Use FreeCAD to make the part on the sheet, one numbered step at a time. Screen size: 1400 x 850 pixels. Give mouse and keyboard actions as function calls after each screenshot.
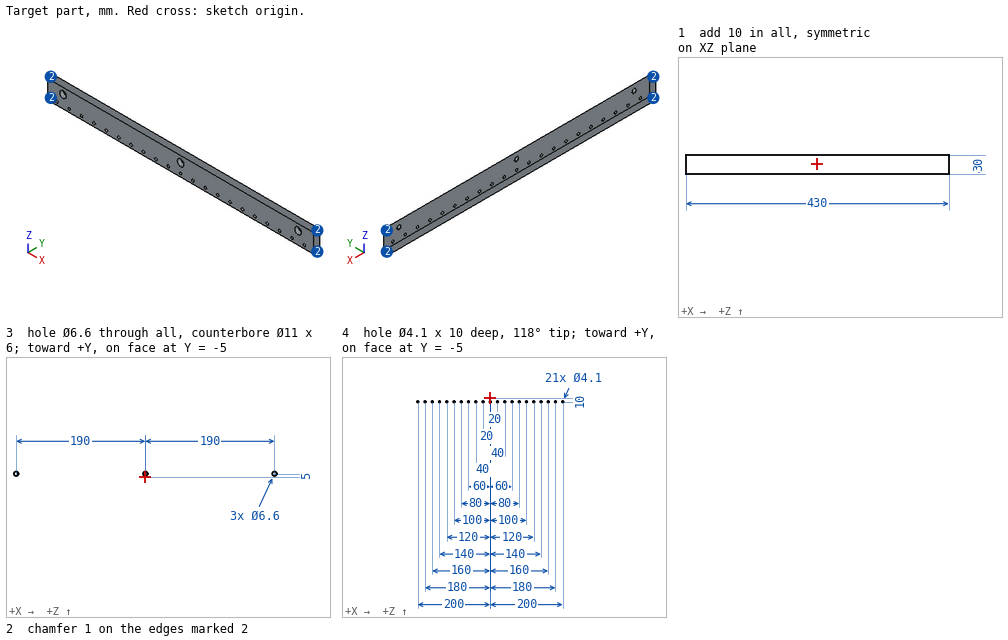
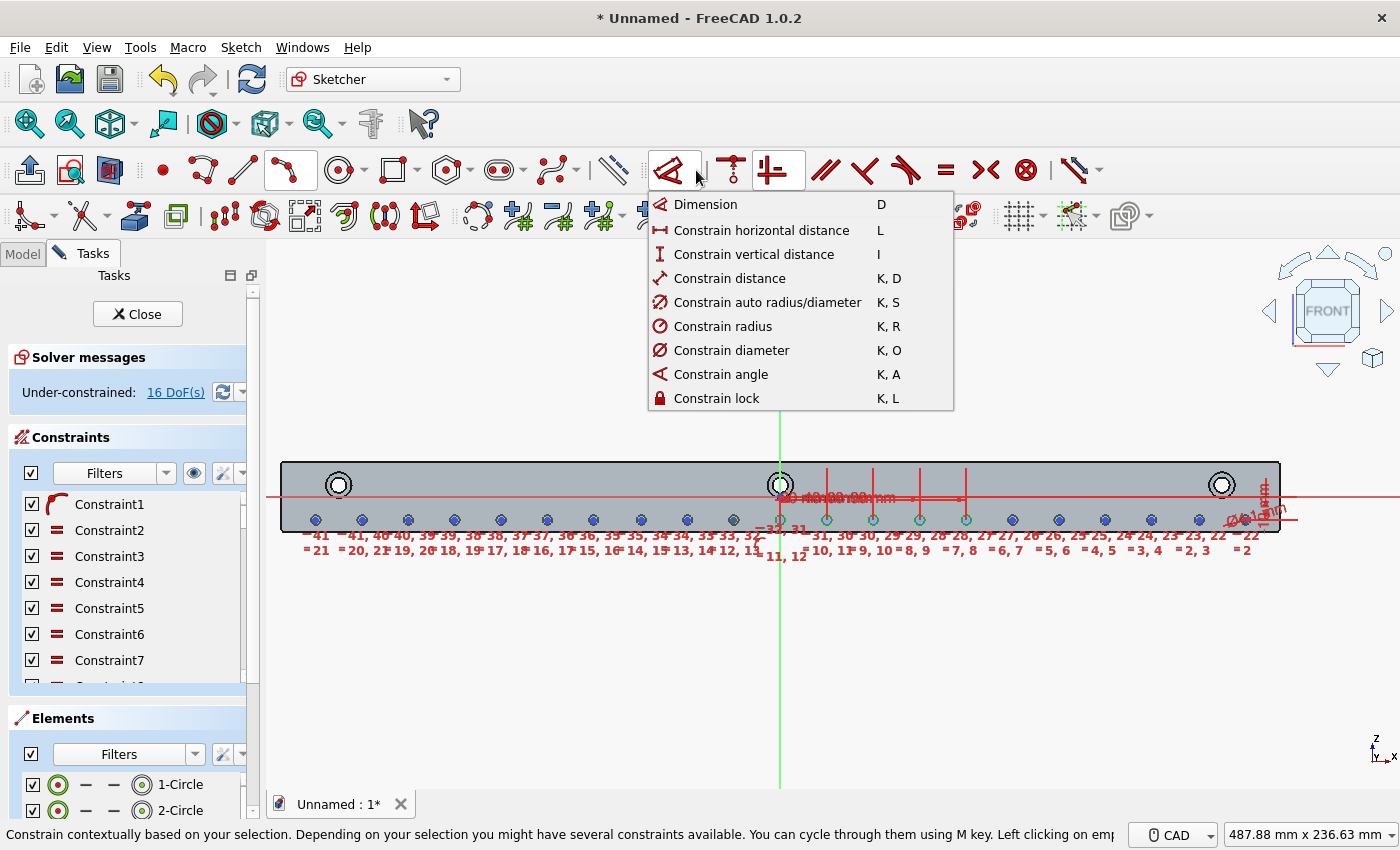
click(801, 230)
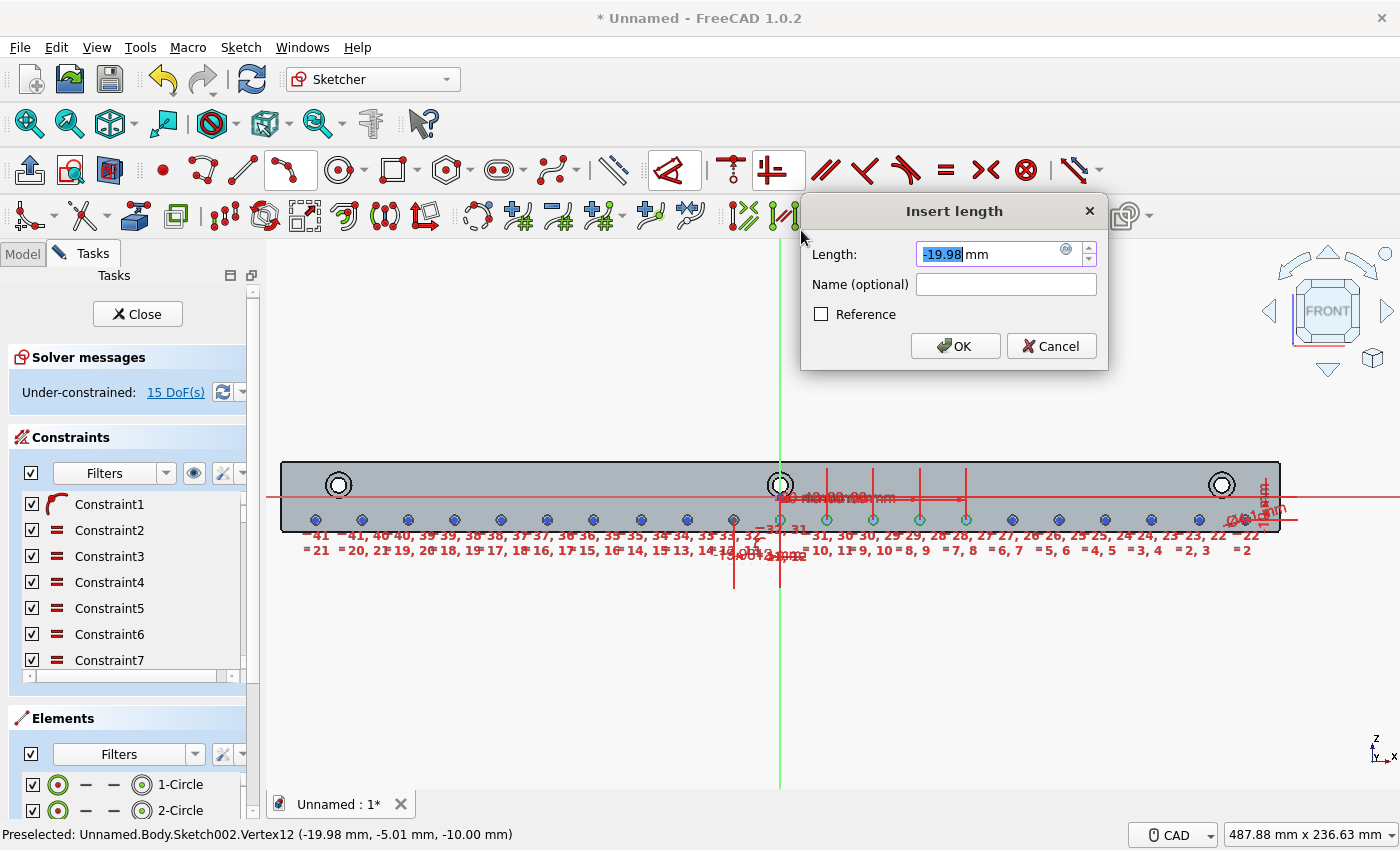
text(-20)
key(Return)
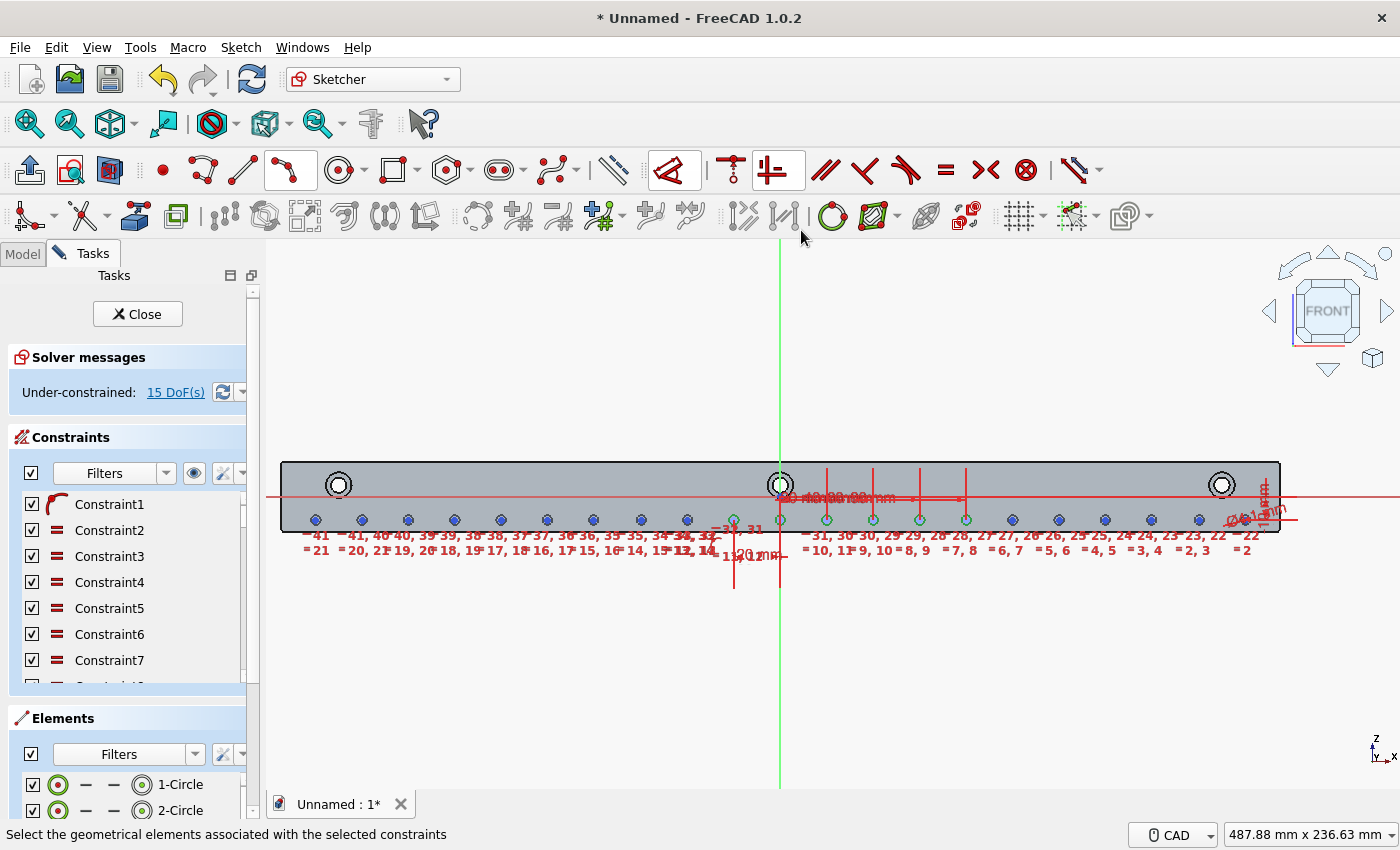
click(688, 520)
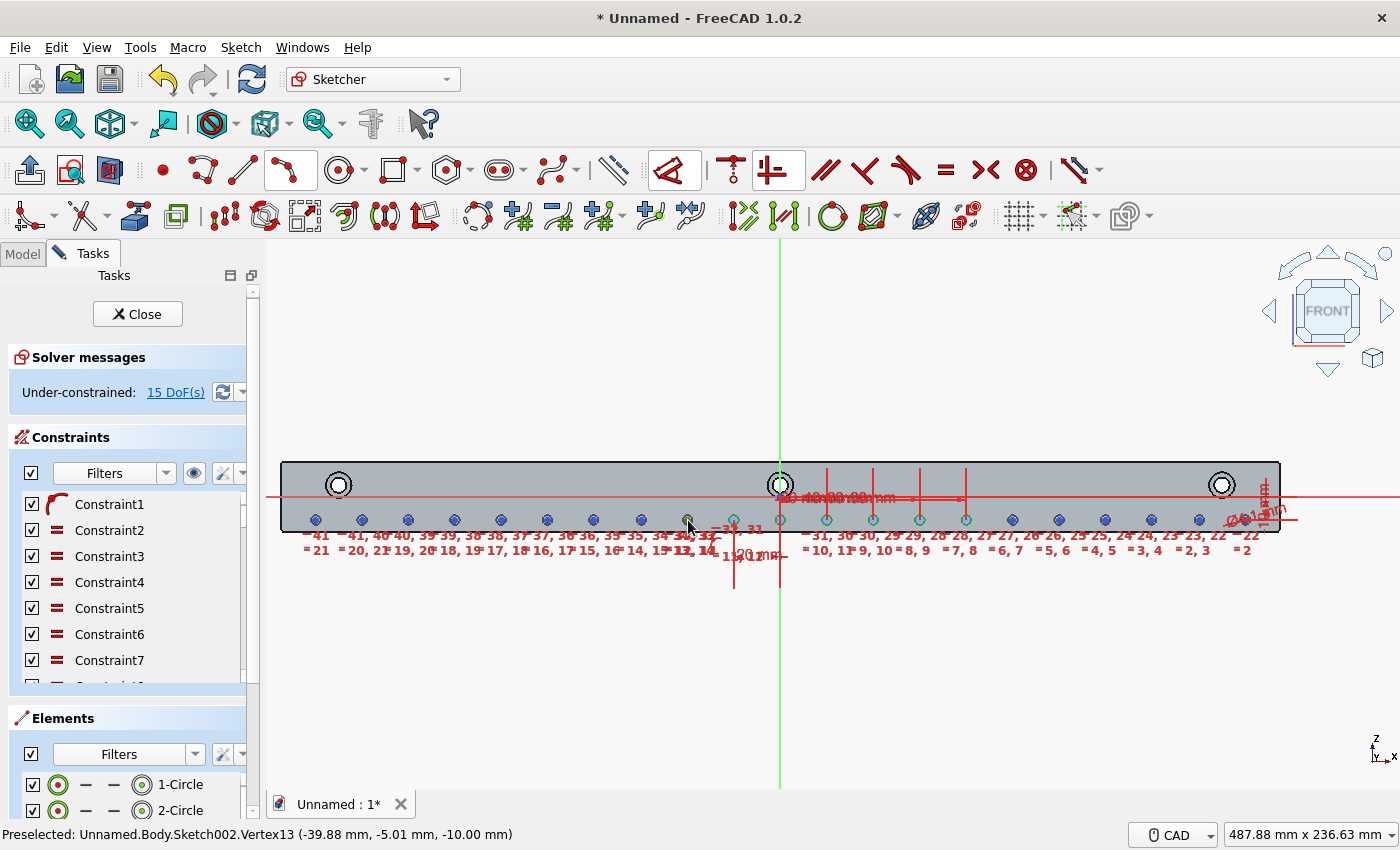
key(l)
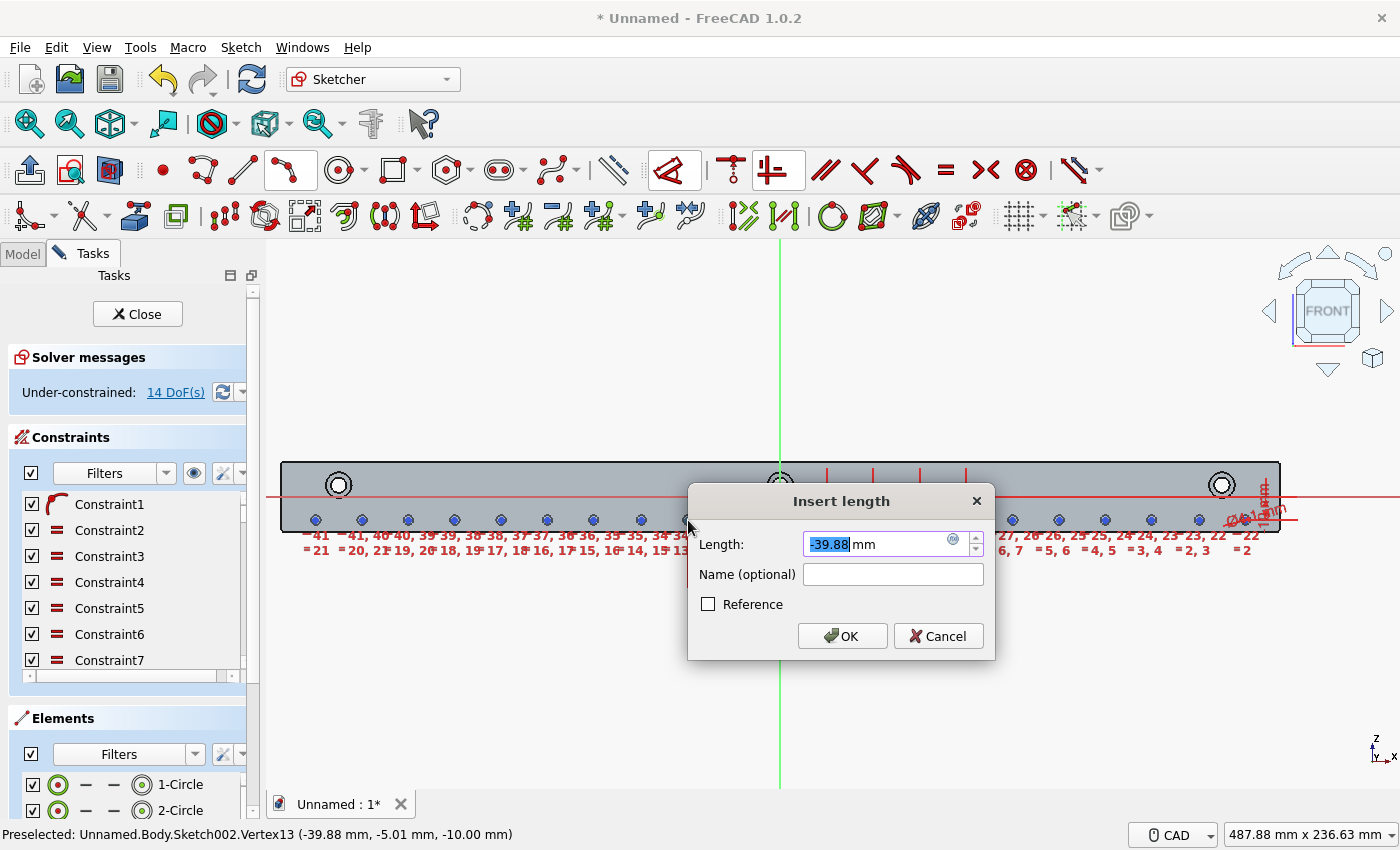
text(-40)
key(Return)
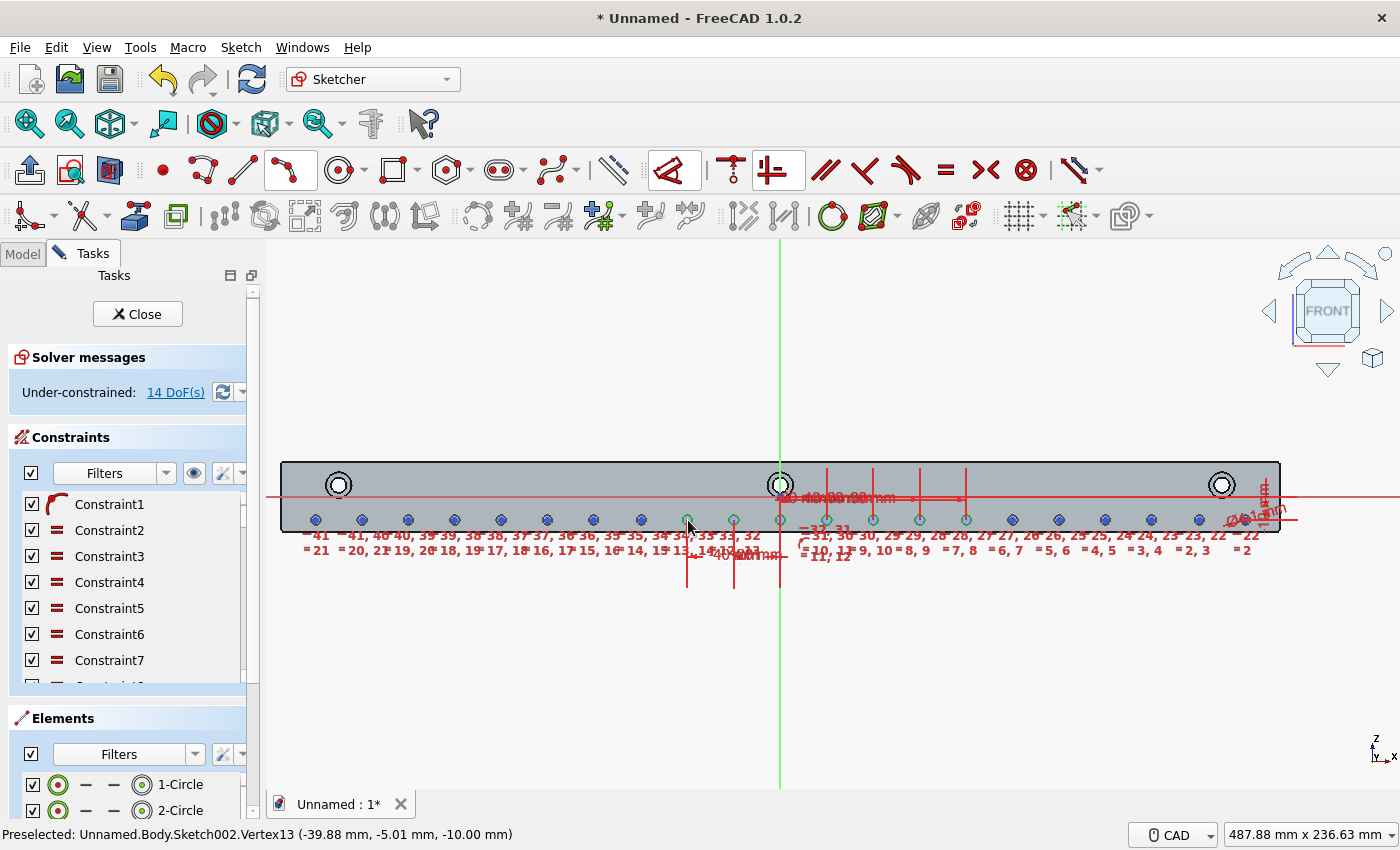
click(641, 520)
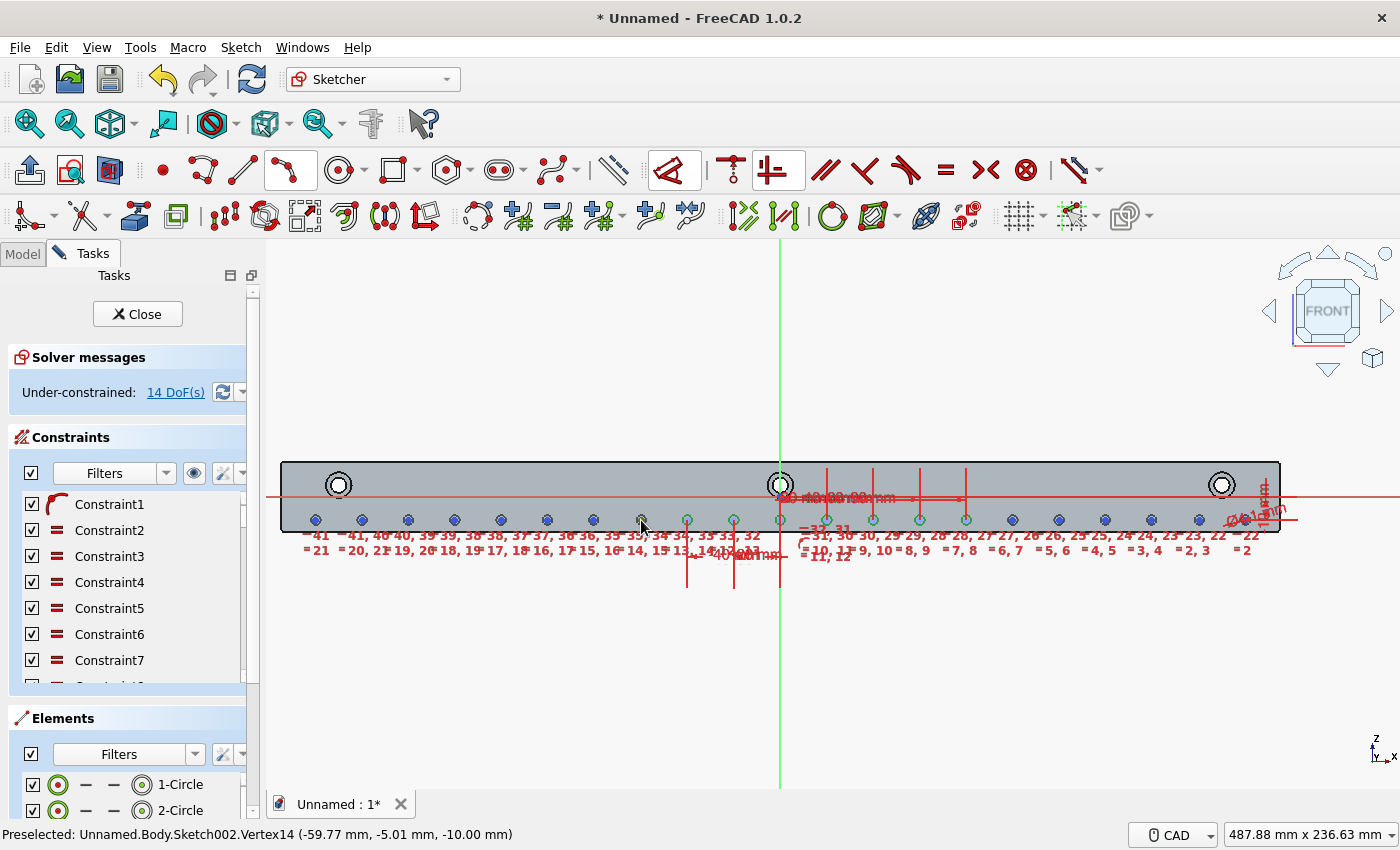
click(696, 170)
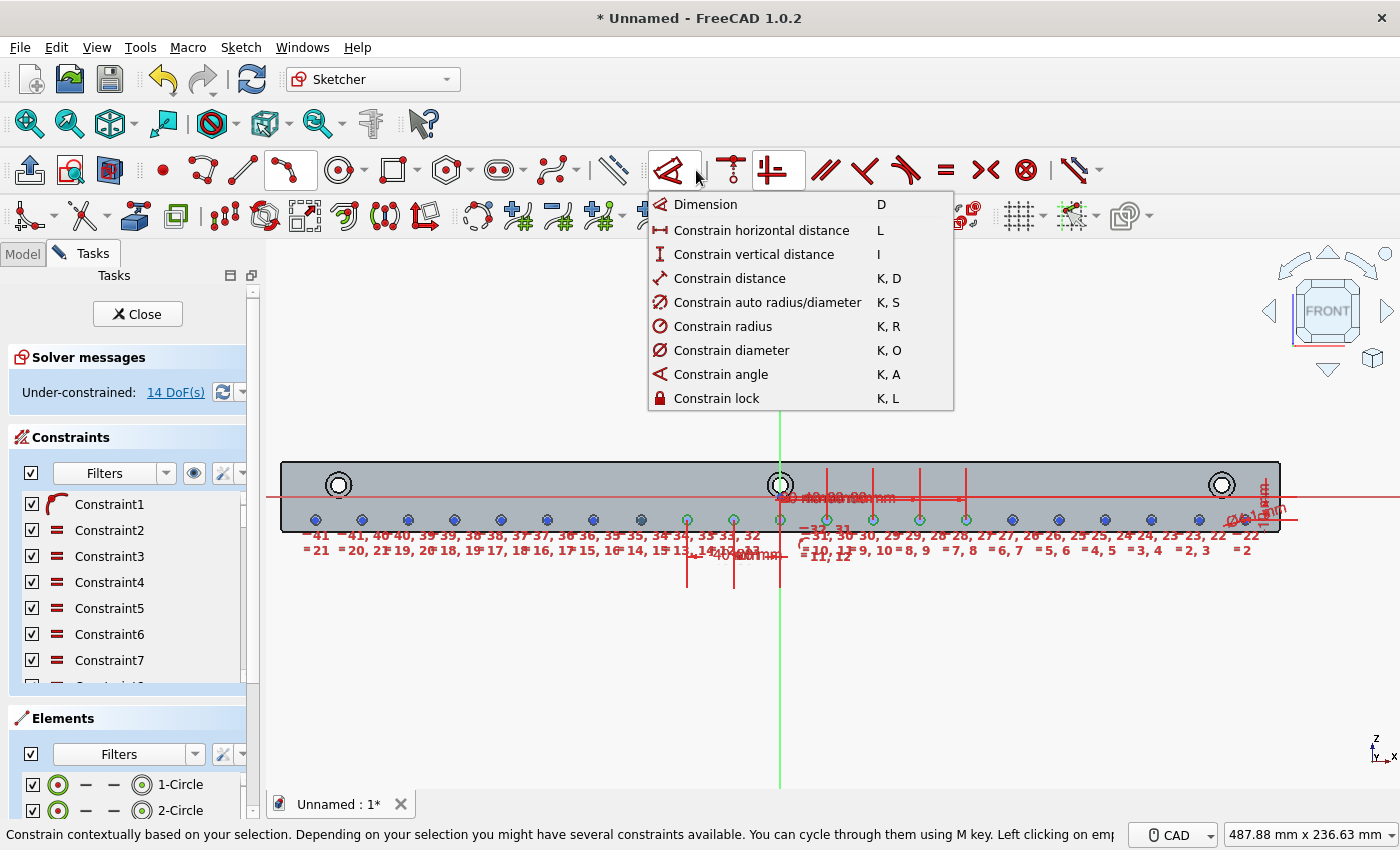
click(801, 230)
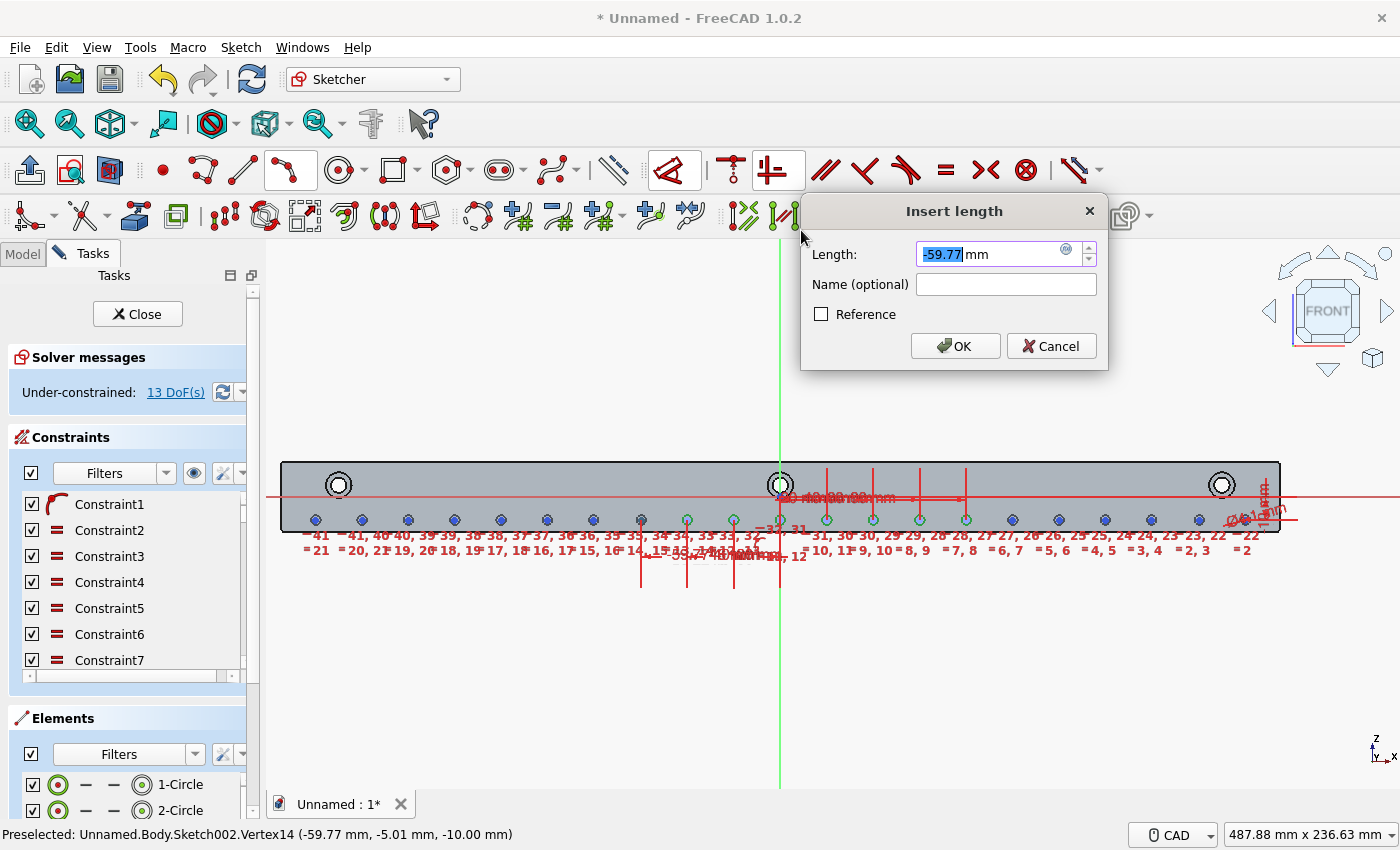
text(-60)
key(Return)